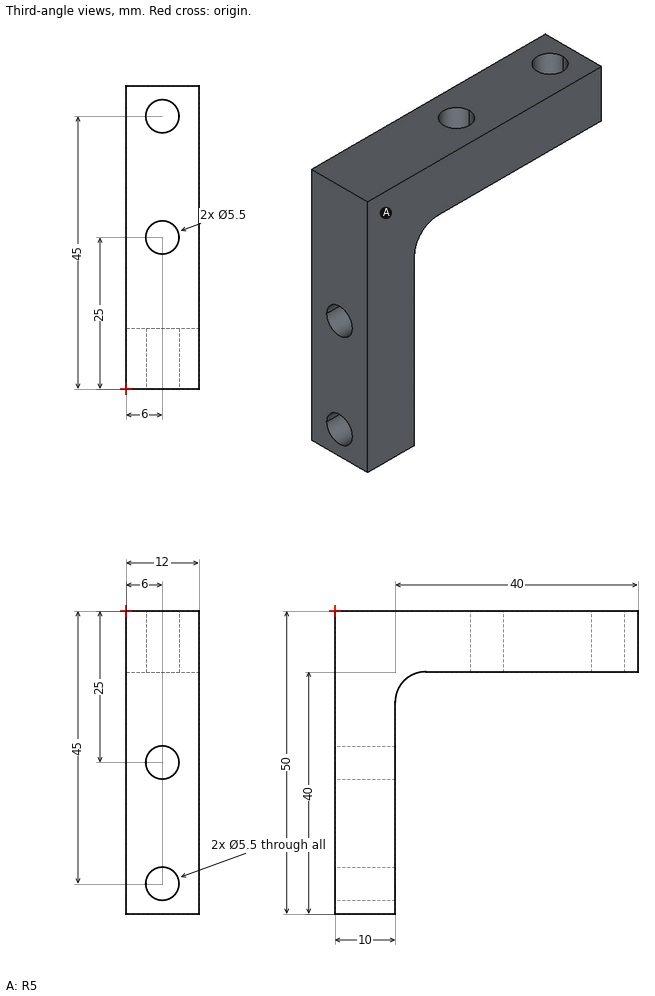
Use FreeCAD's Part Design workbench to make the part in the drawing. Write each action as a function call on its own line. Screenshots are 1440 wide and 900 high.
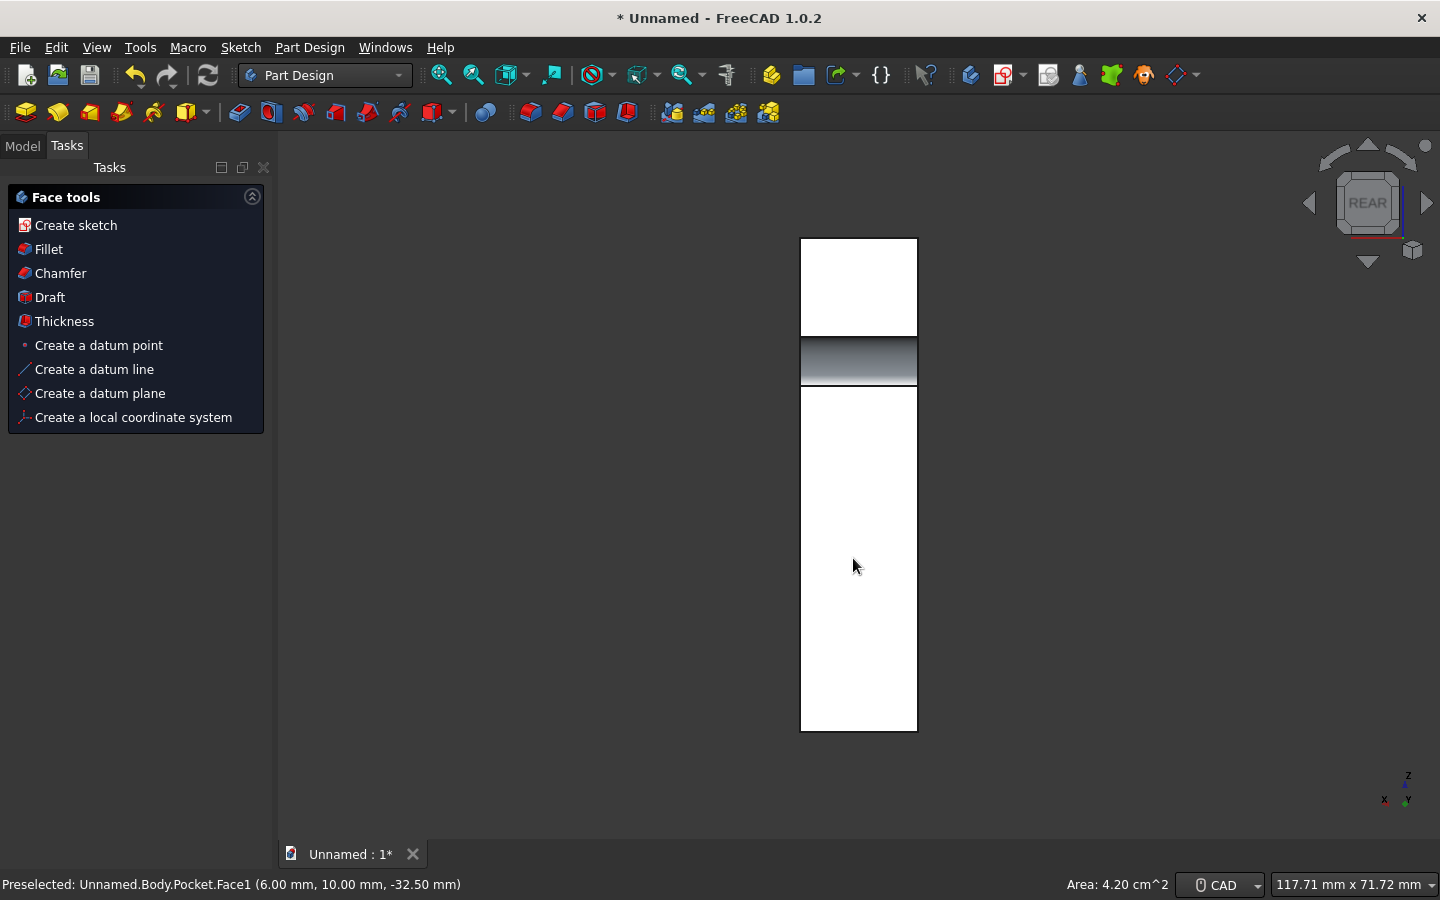
click(1004, 76)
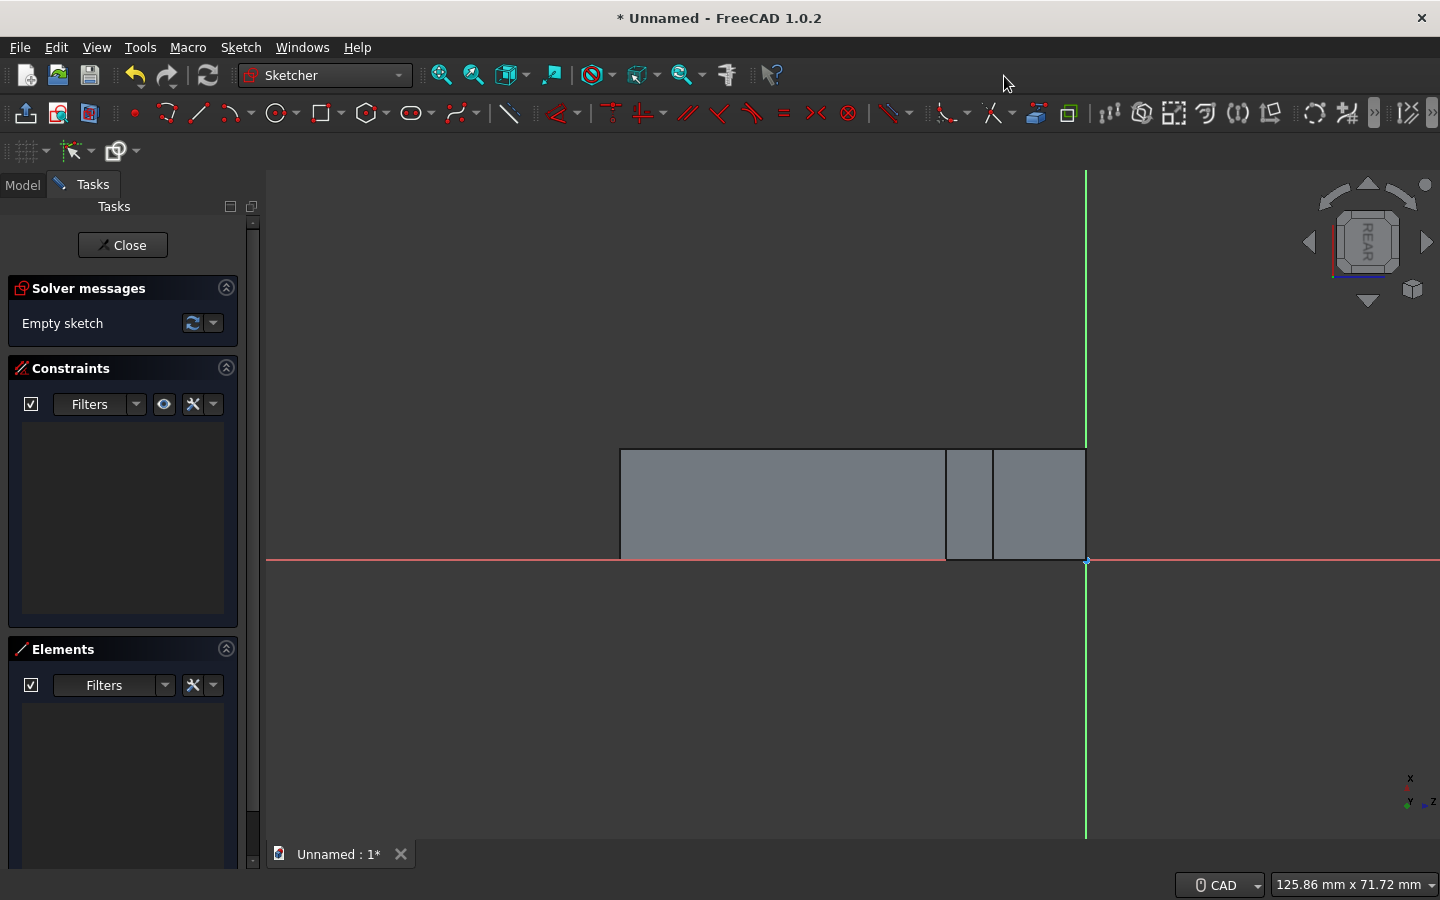
scroll(1024, 550, up, 2)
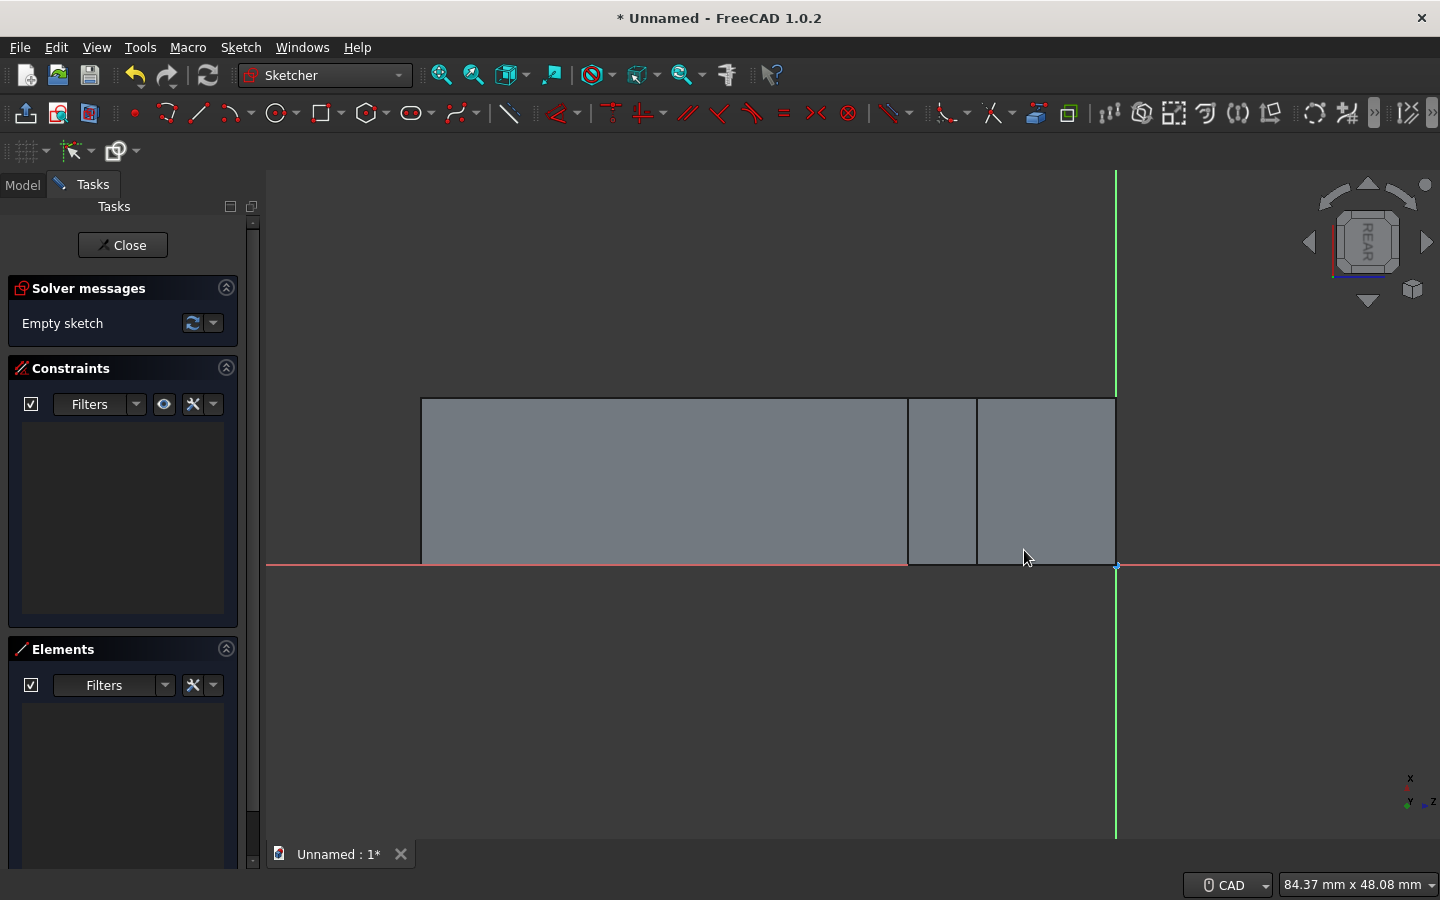
click(276, 114)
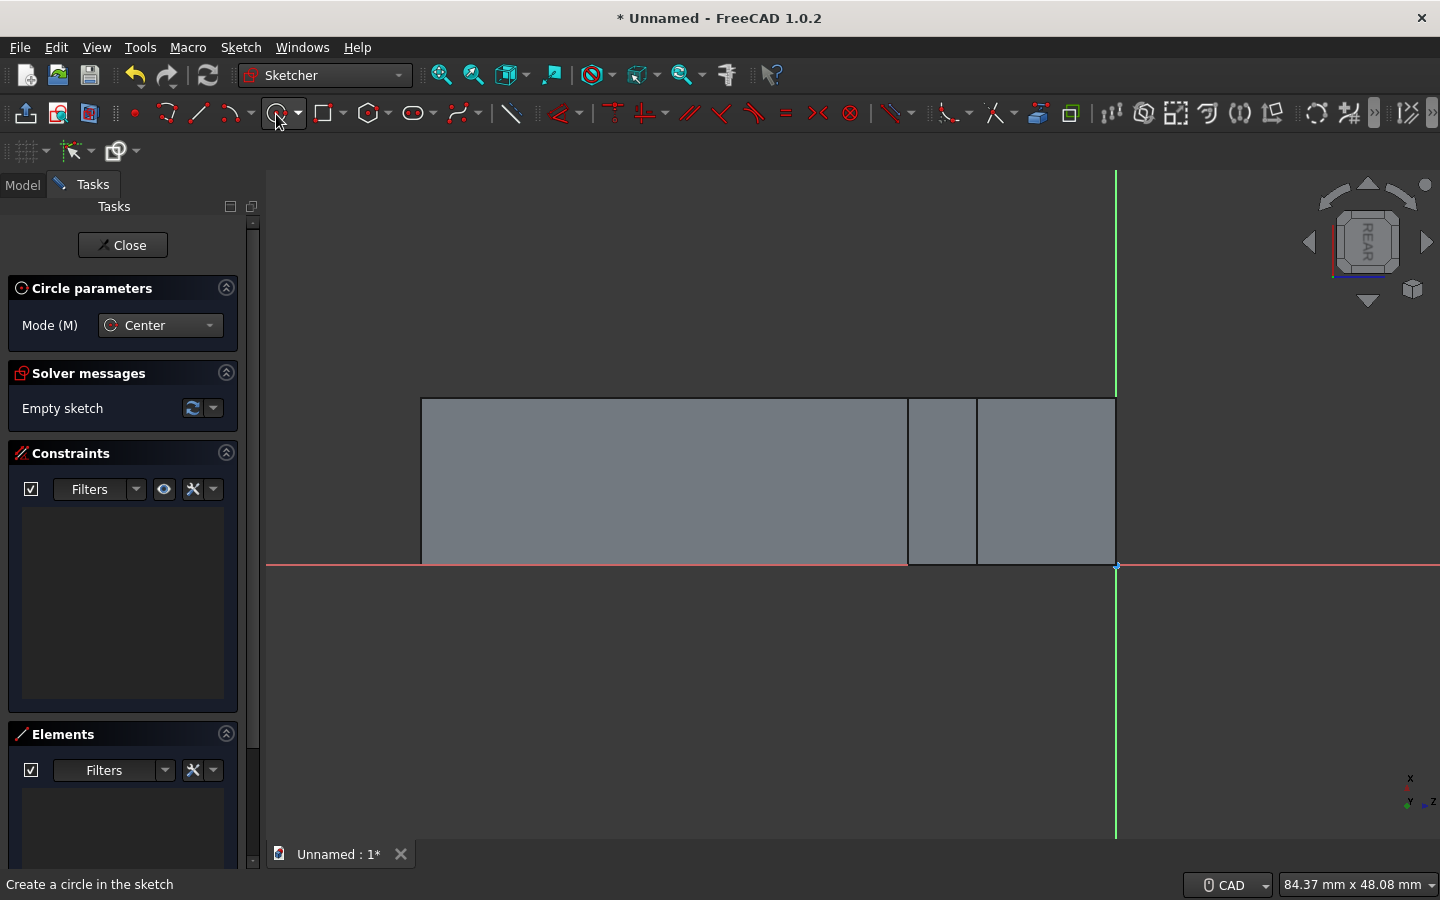
click(490, 482)
click(517, 455)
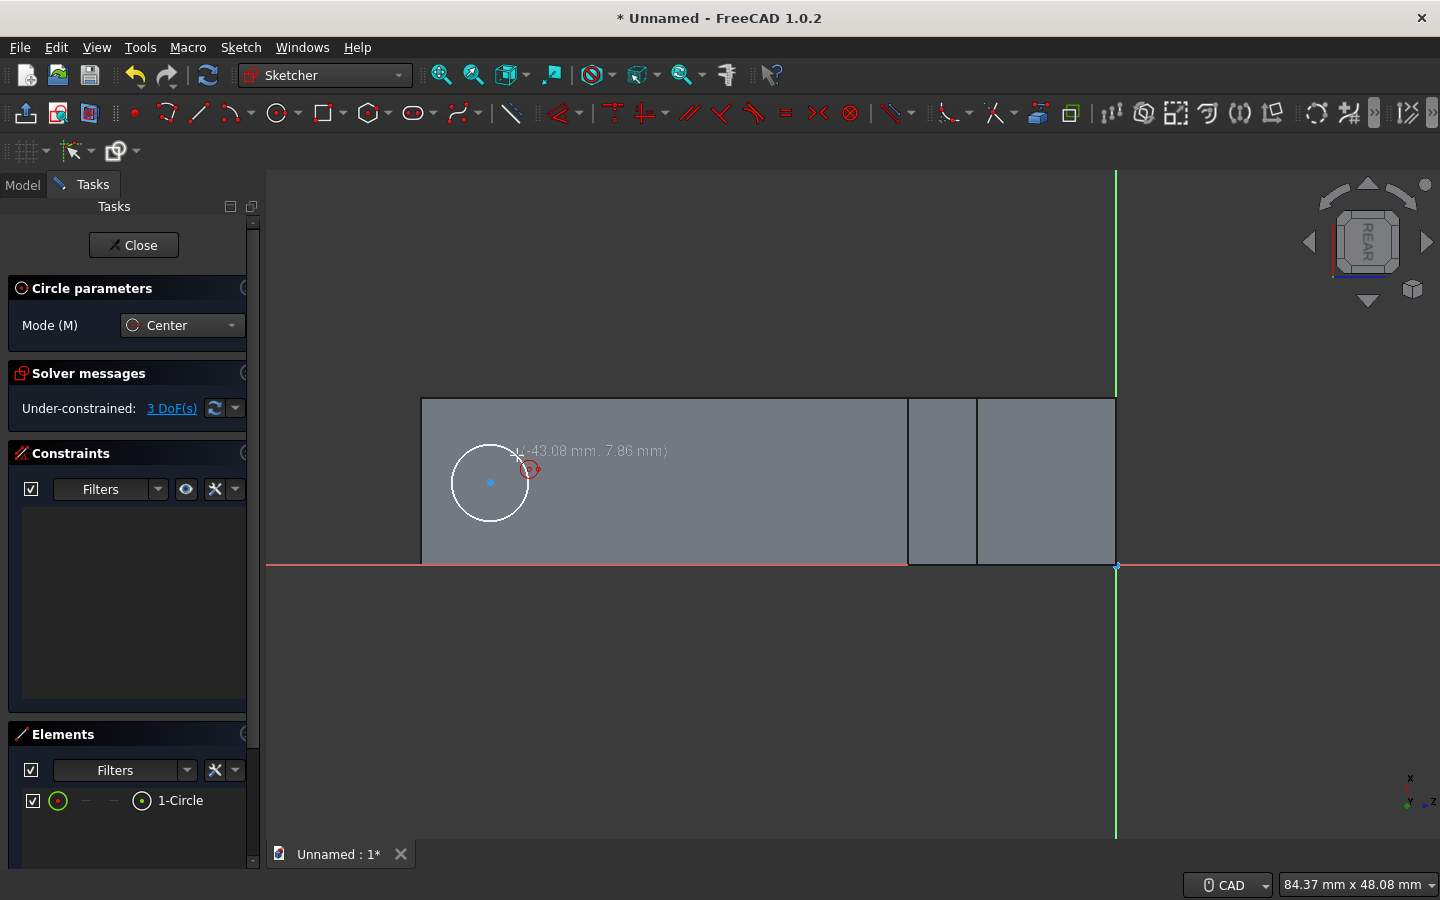
click(769, 482)
click(796, 455)
key(Escape)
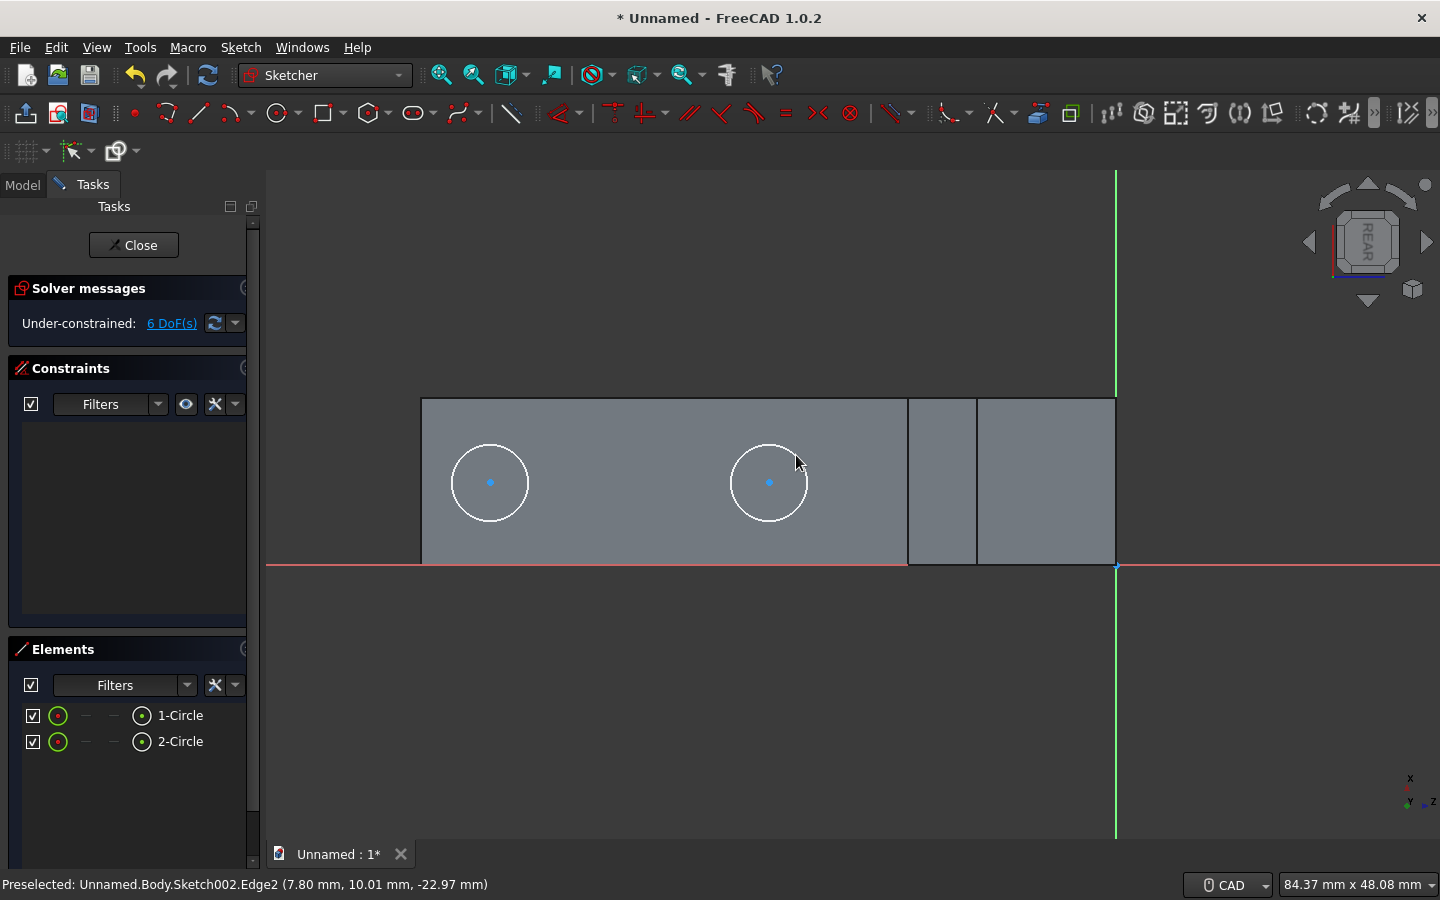
click(517, 456)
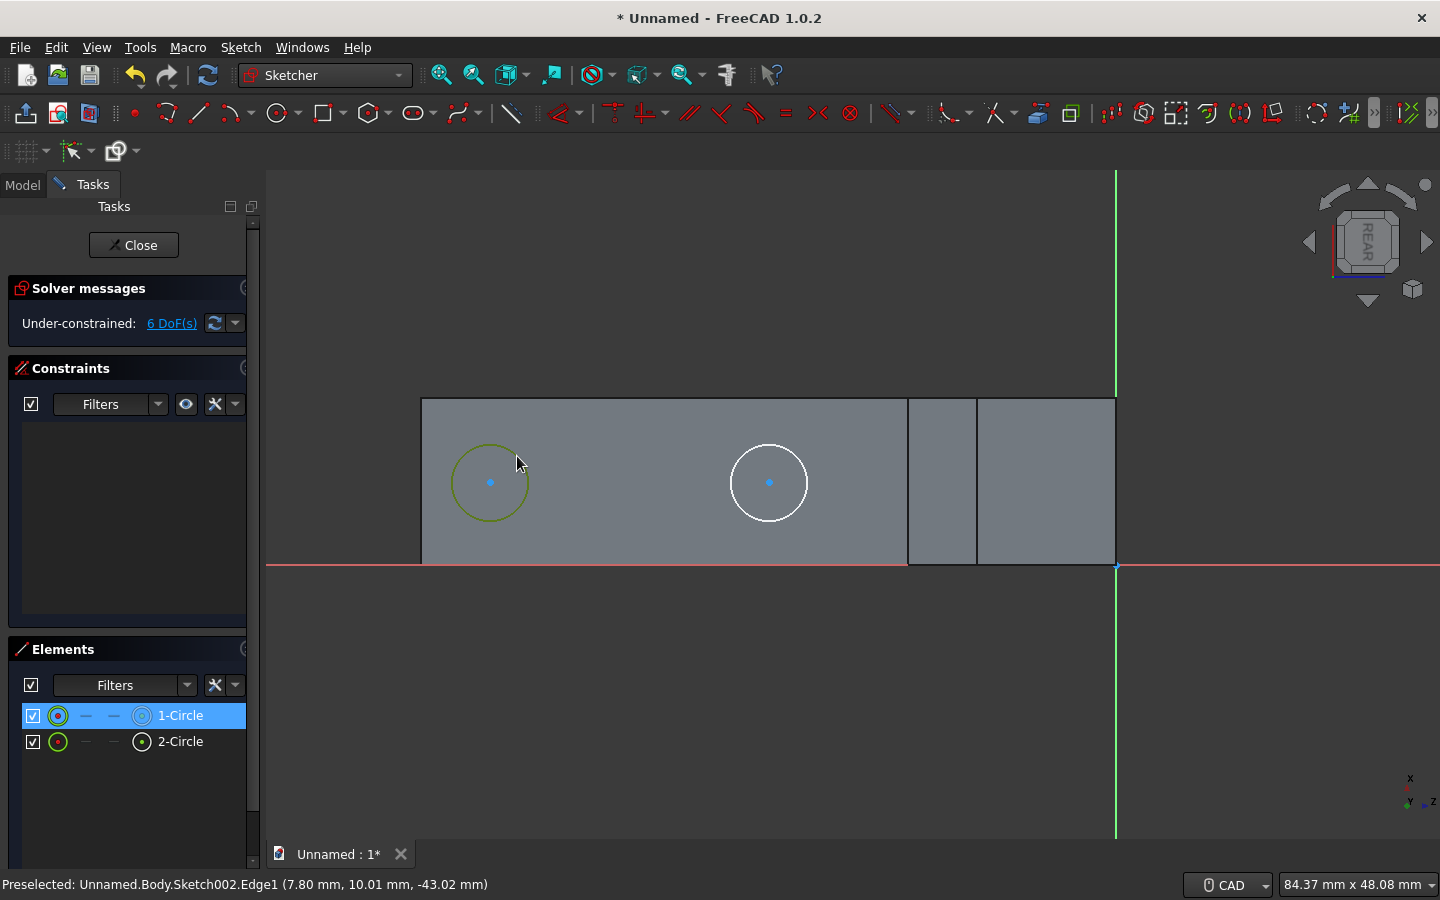
click(796, 456)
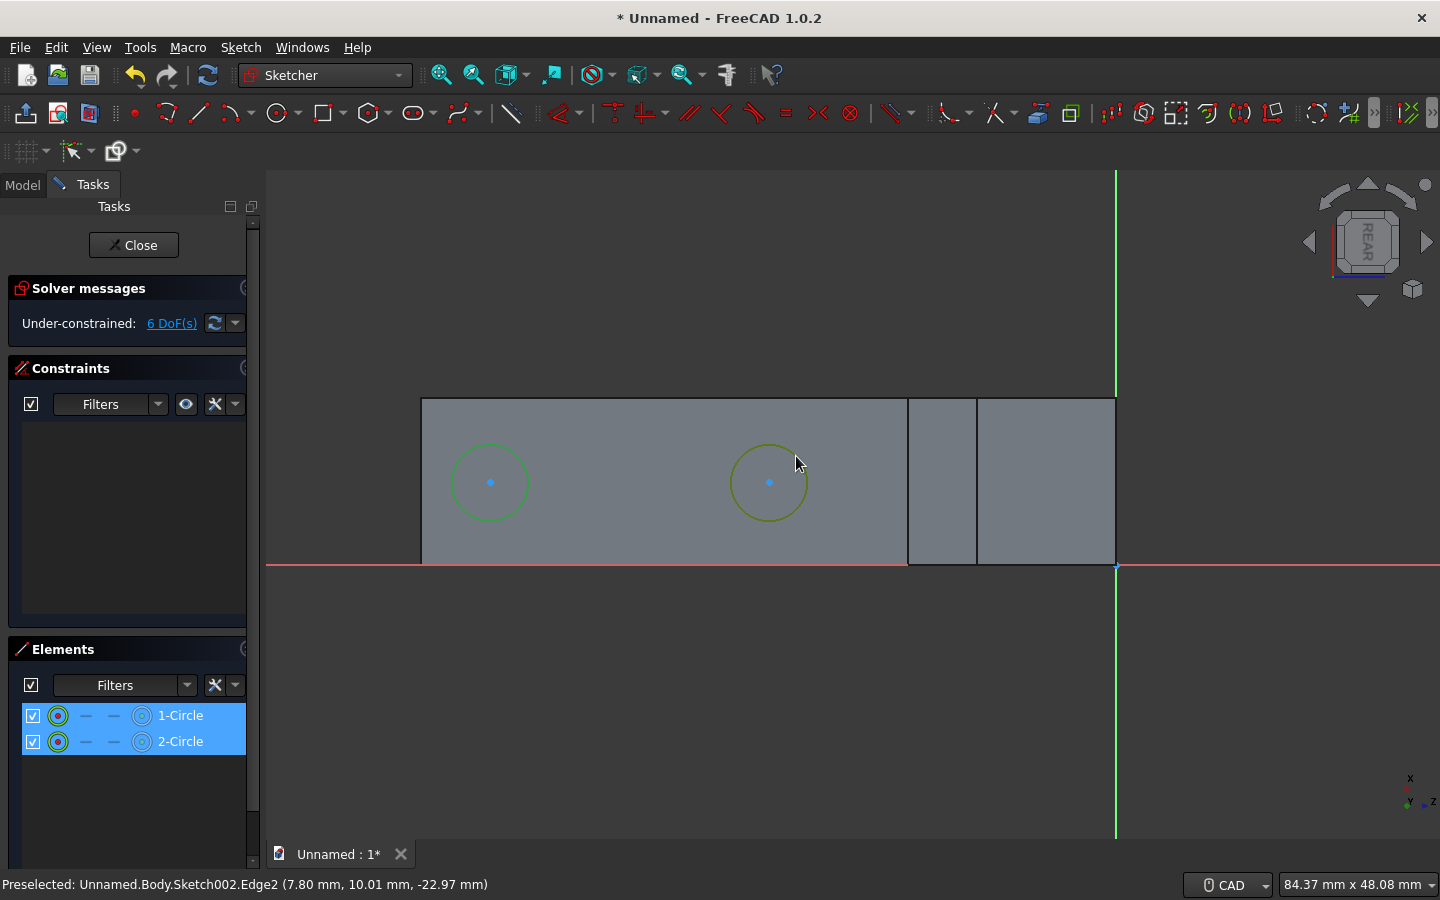
click(786, 114)